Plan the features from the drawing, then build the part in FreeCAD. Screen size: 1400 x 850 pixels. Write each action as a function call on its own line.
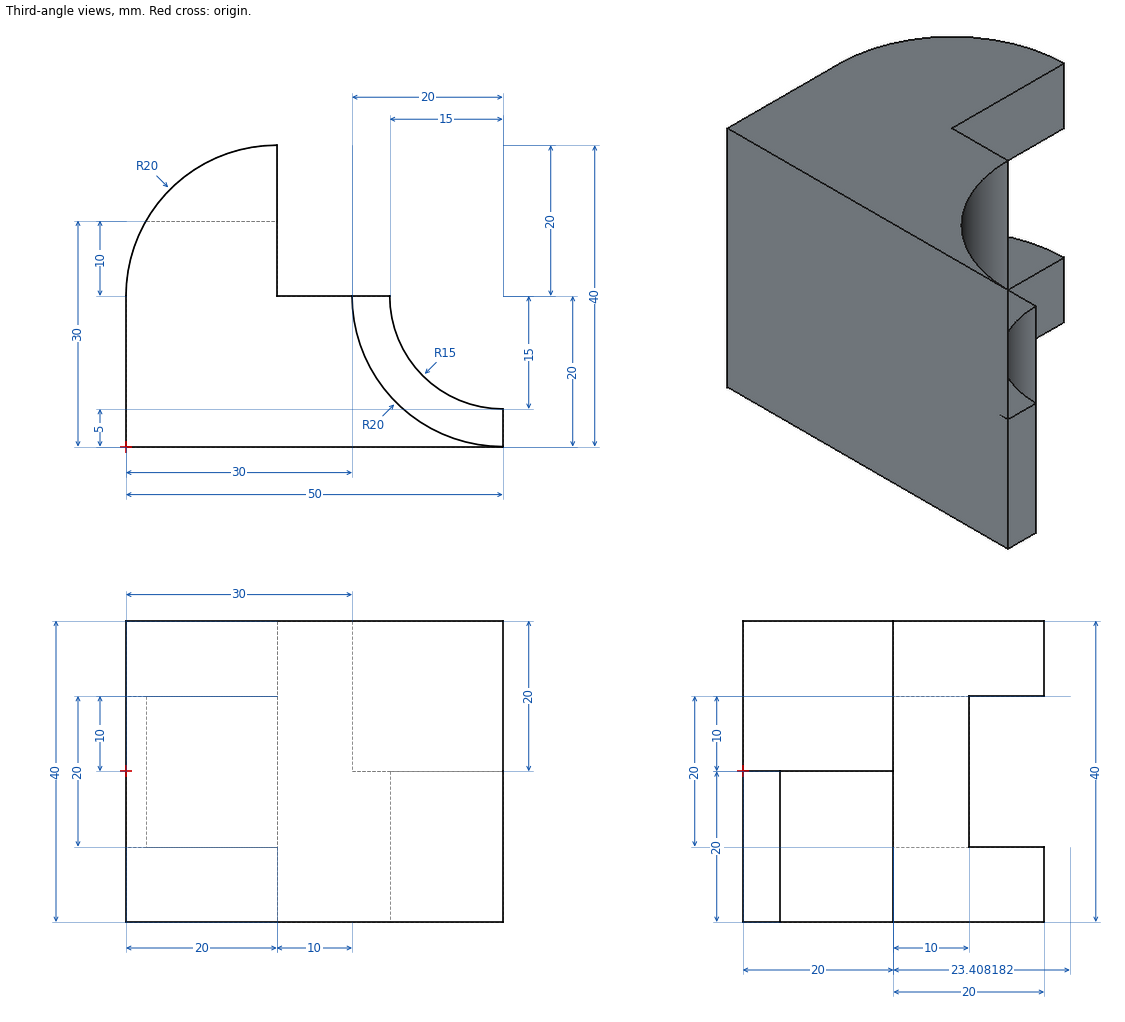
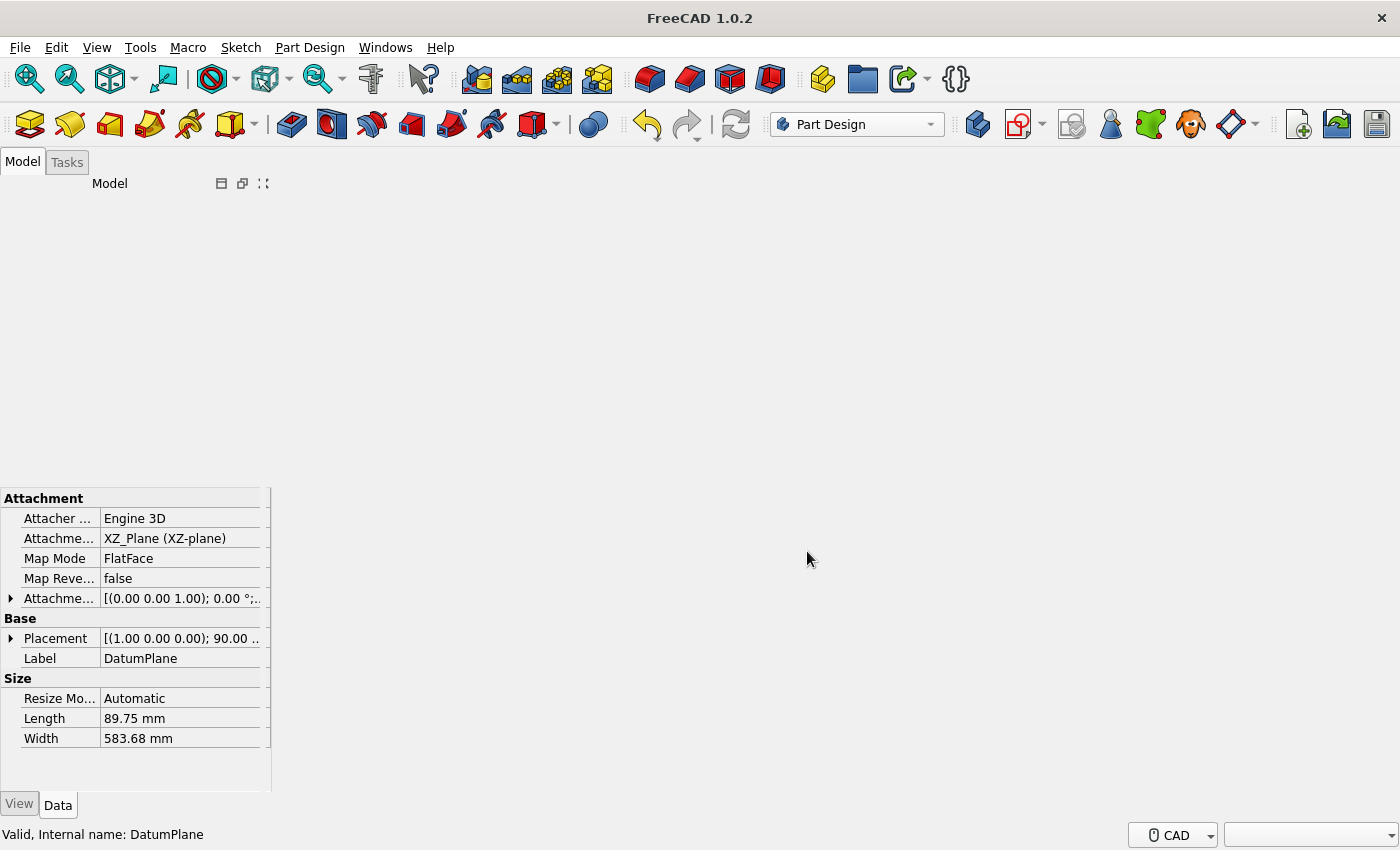
key(ctrl+n)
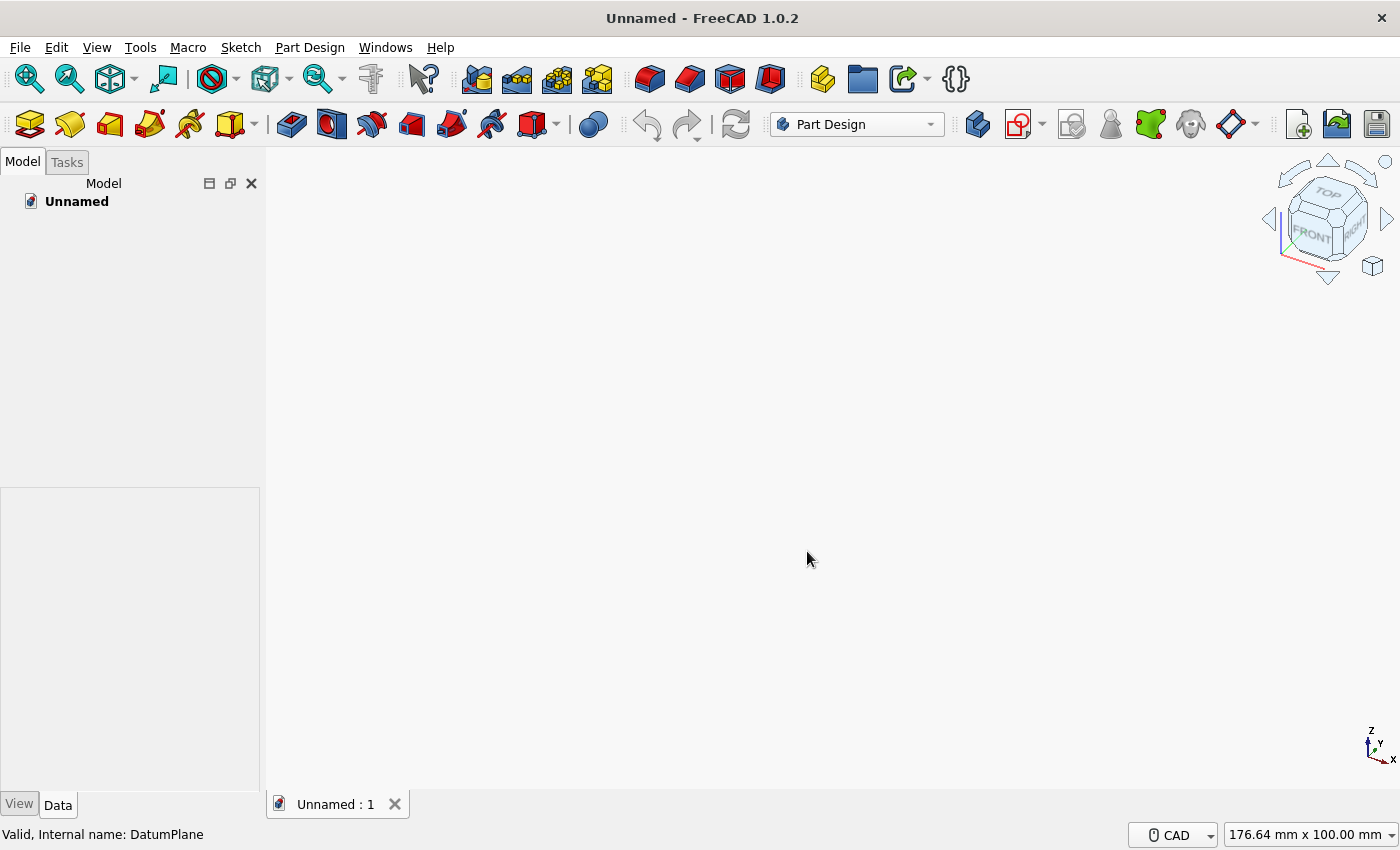
click(1018, 124)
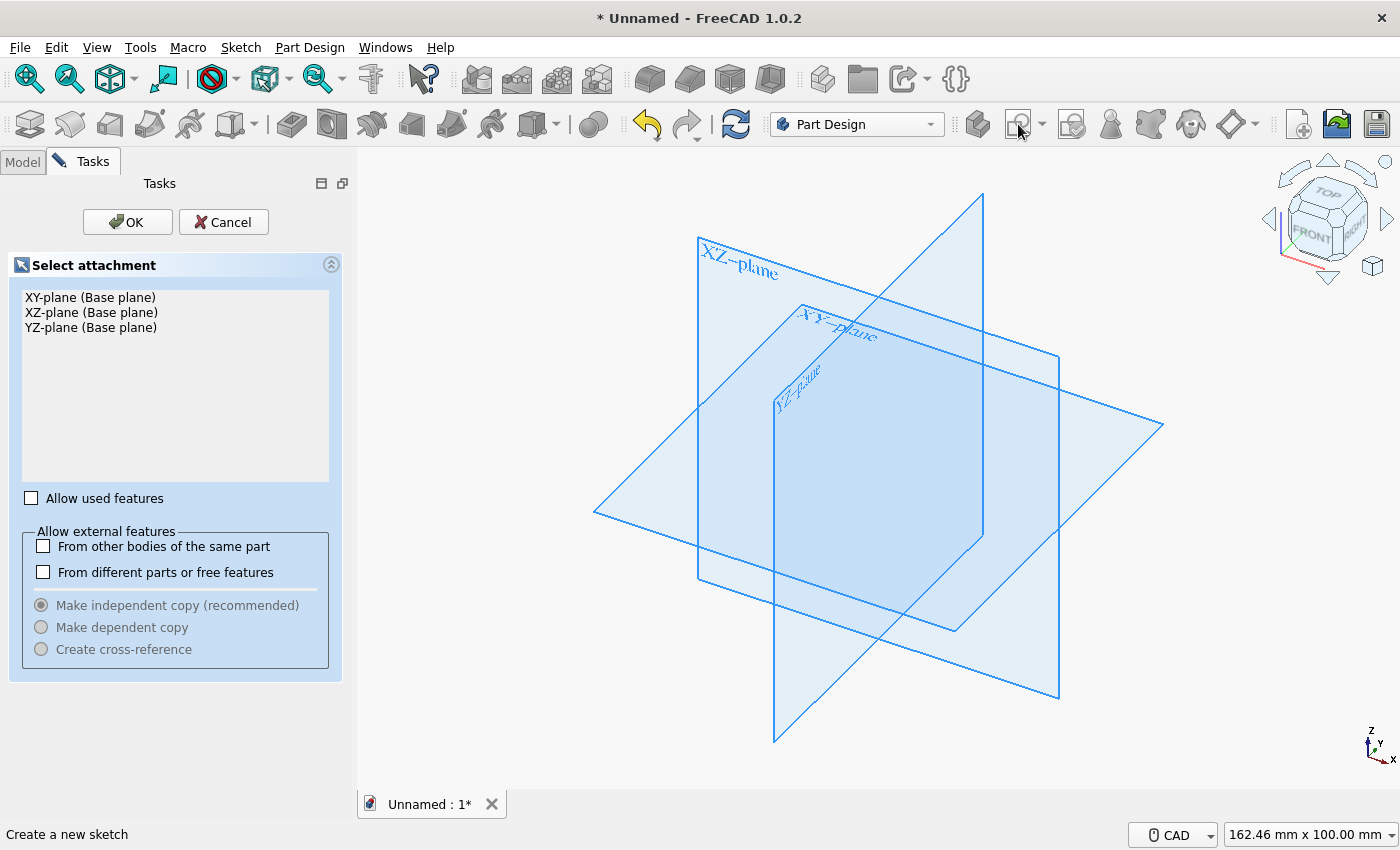
click(82, 298)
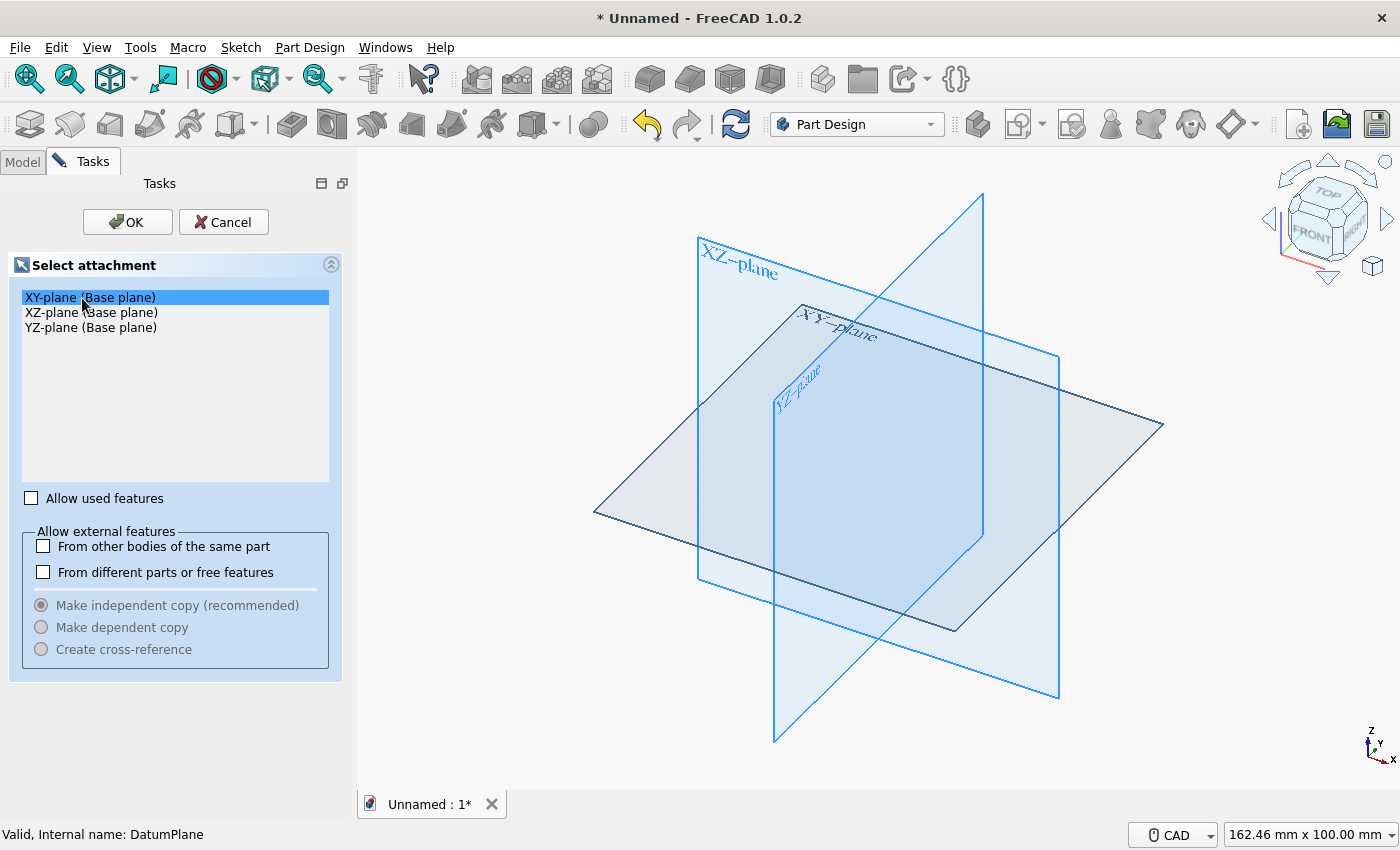
click(128, 222)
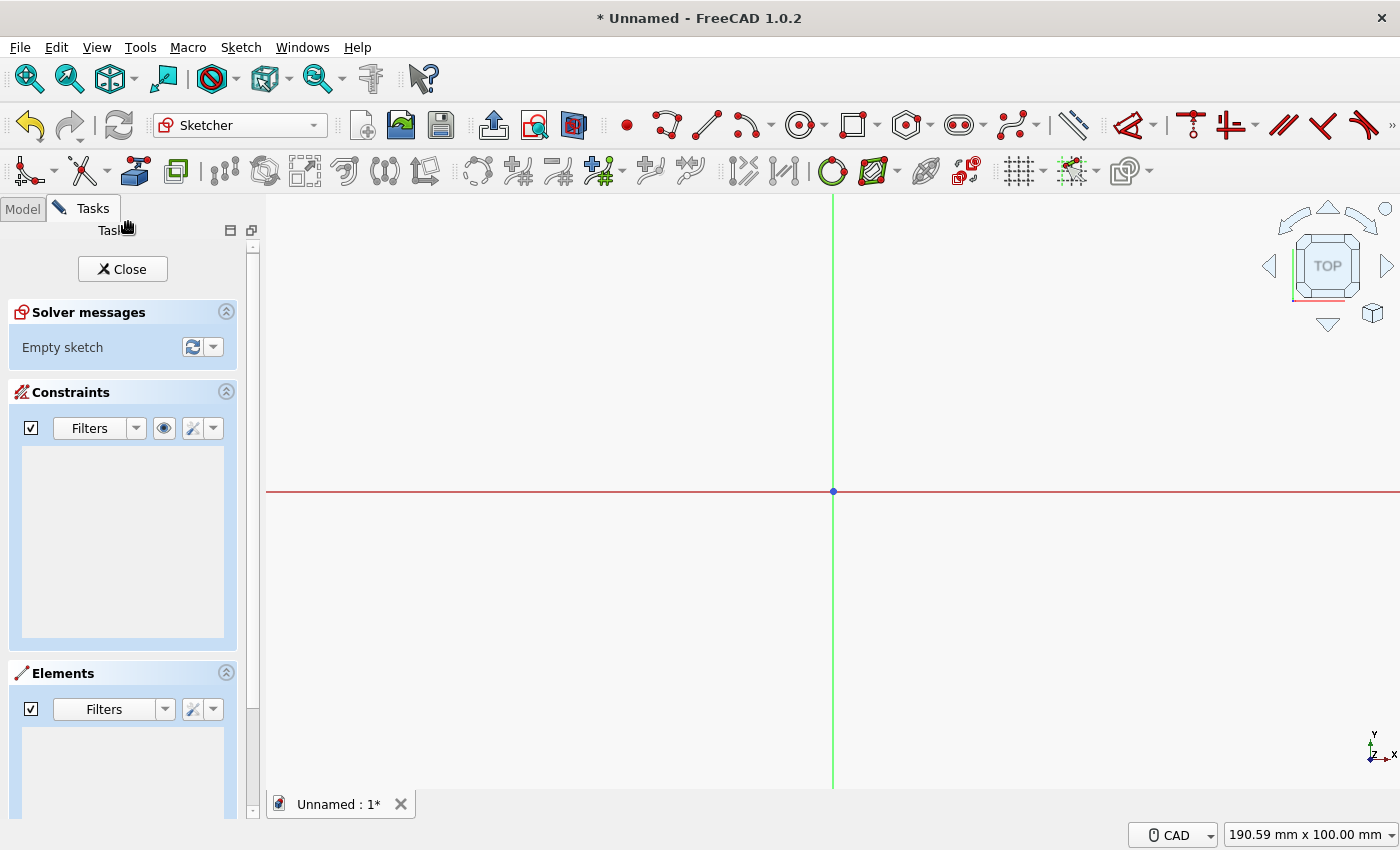
scroll(1235, 222, up, 2)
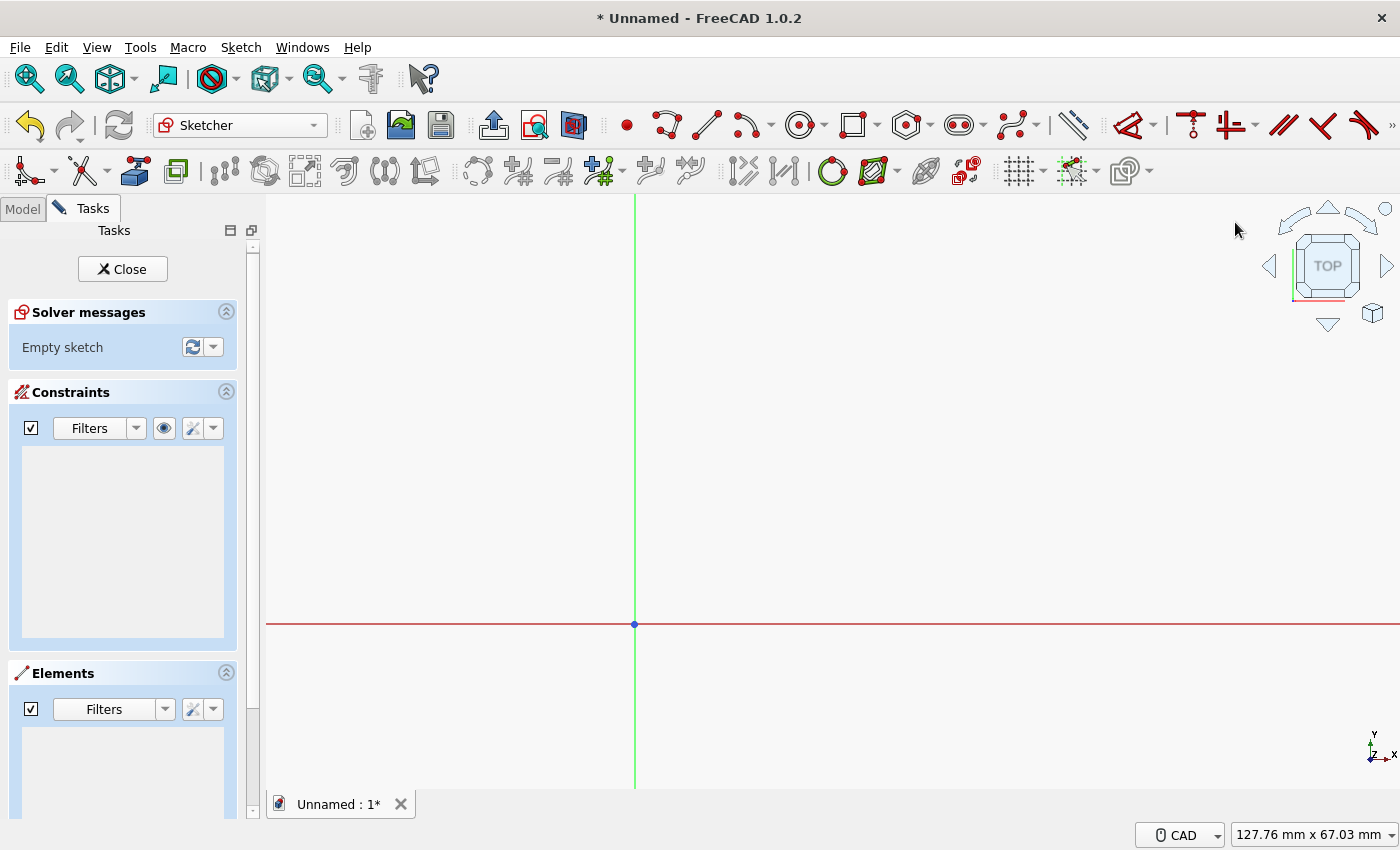
click(854, 126)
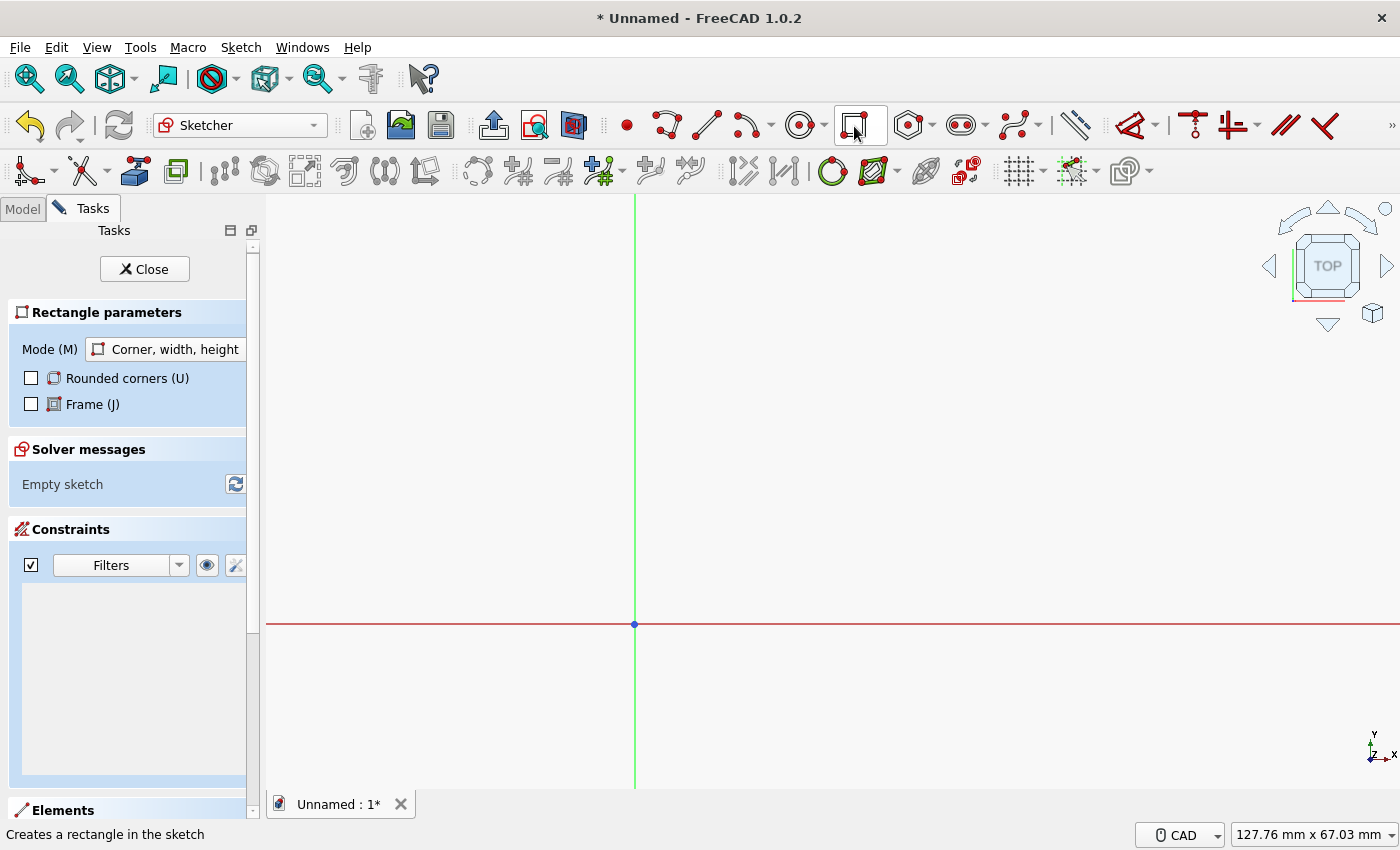
click(635, 624)
move(1079, 269)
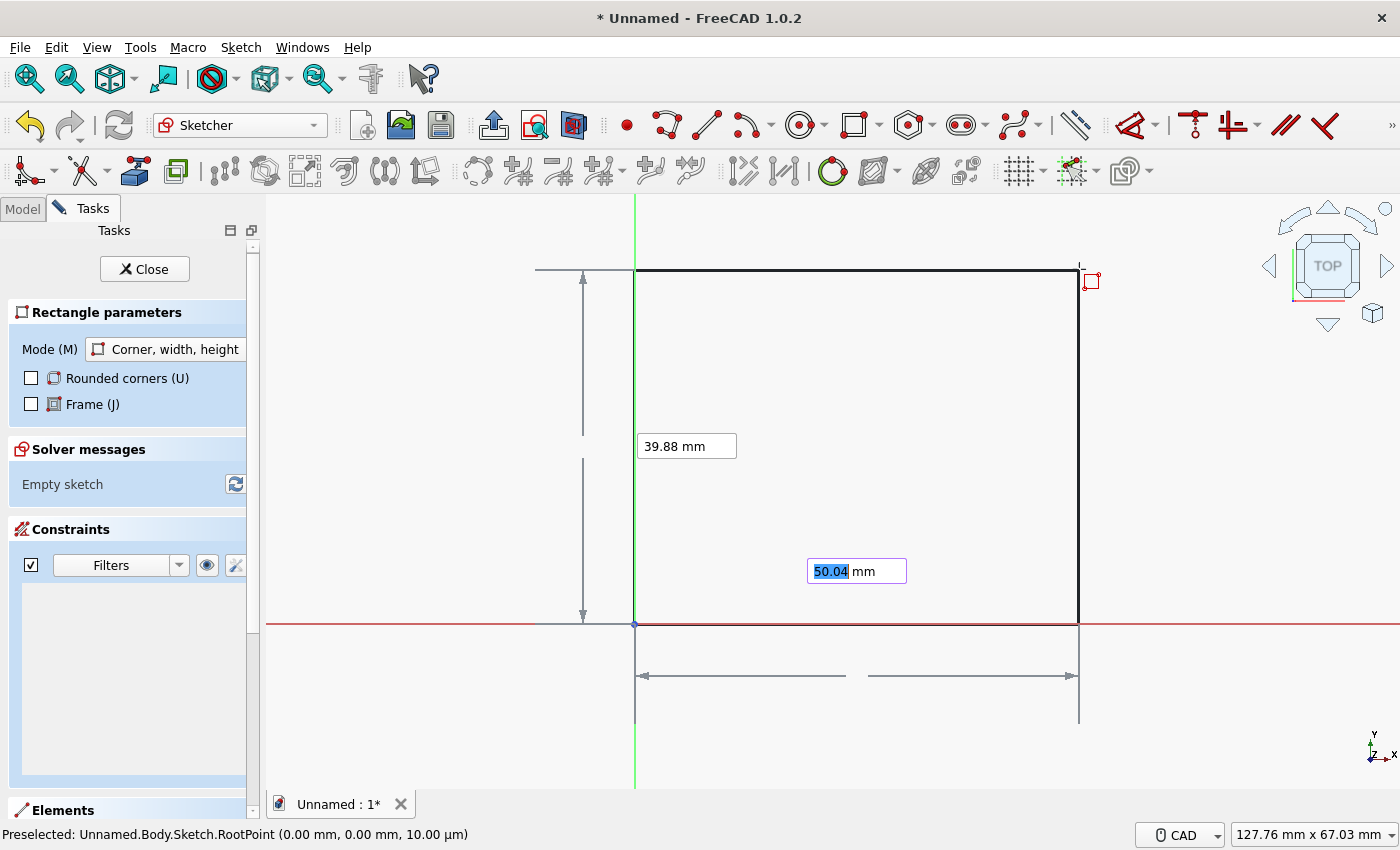
text(50)
key(Tab)
text(40)
key(Return)
key(Escape)